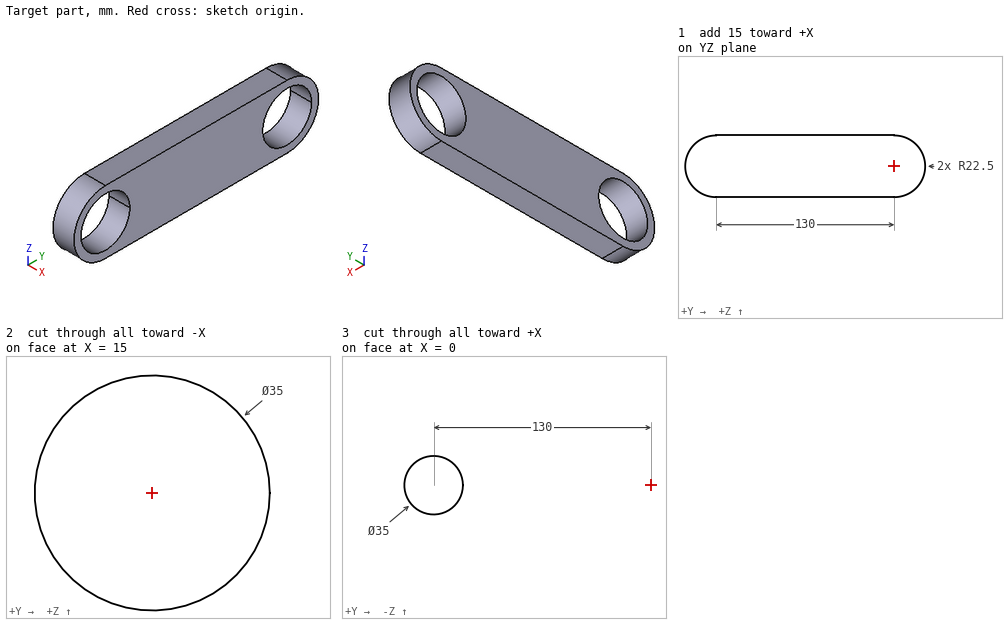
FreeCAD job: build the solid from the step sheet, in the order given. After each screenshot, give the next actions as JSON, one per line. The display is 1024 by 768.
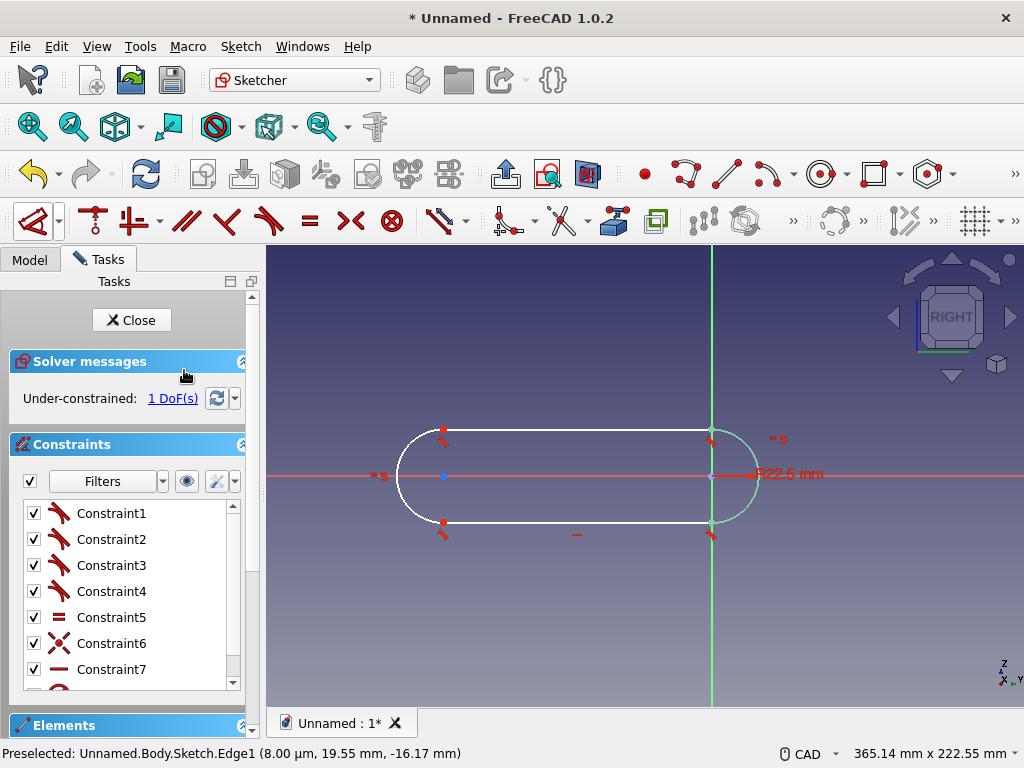
{"action": "left_click", "coordinate": [631, 523]}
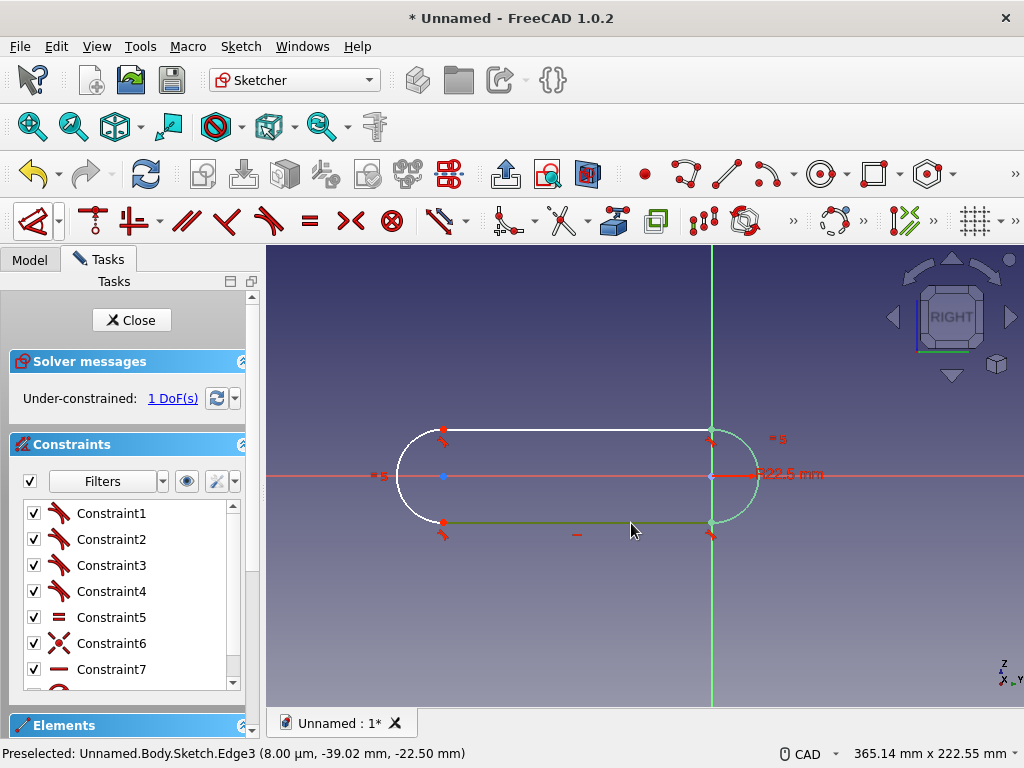
{"action": "left_click", "coordinate": [58, 222]}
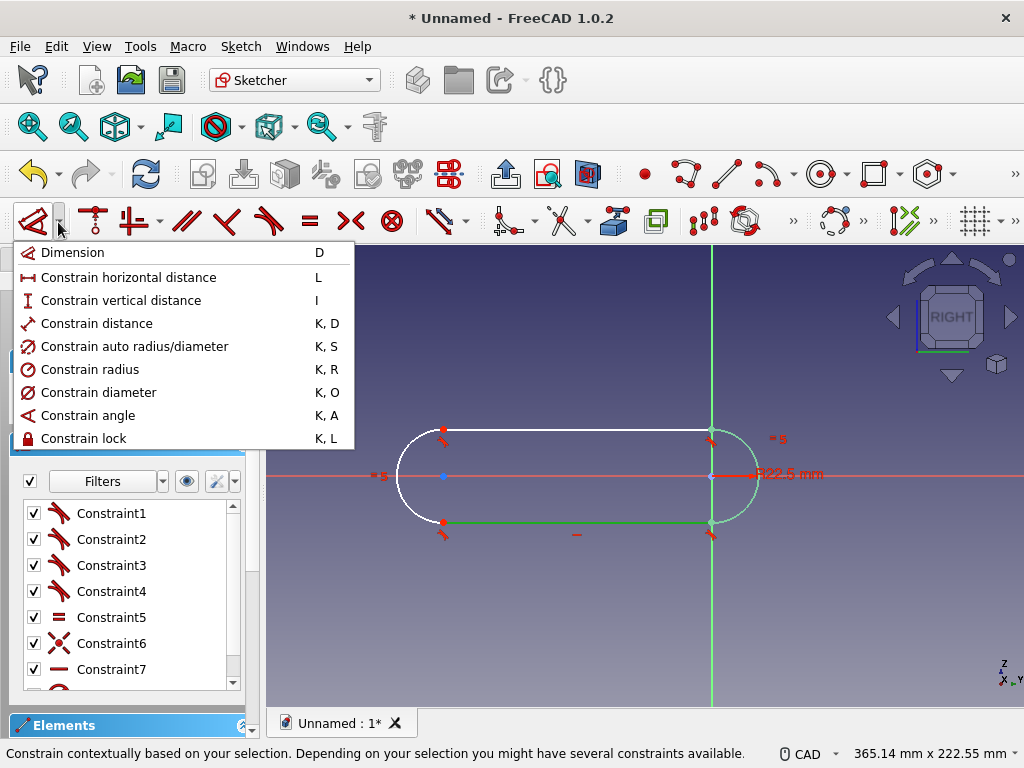
{"action": "left_click", "coordinate": [184, 278]}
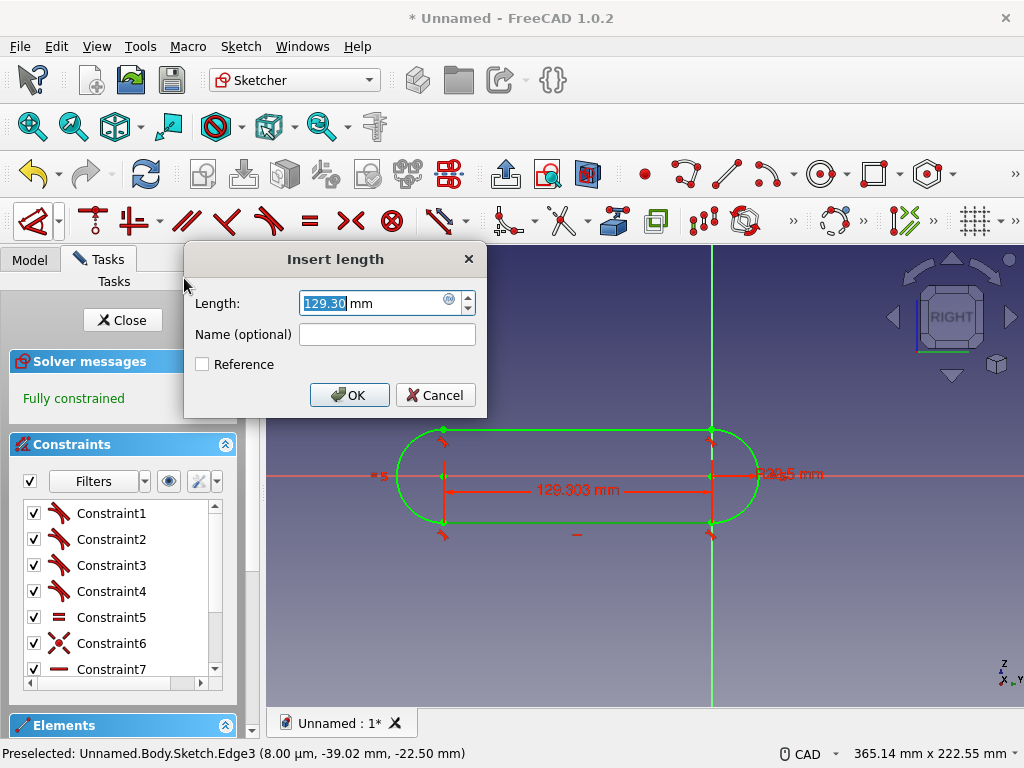
{"action": "type", "text": "130"}
{"action": "key", "text": "Return"}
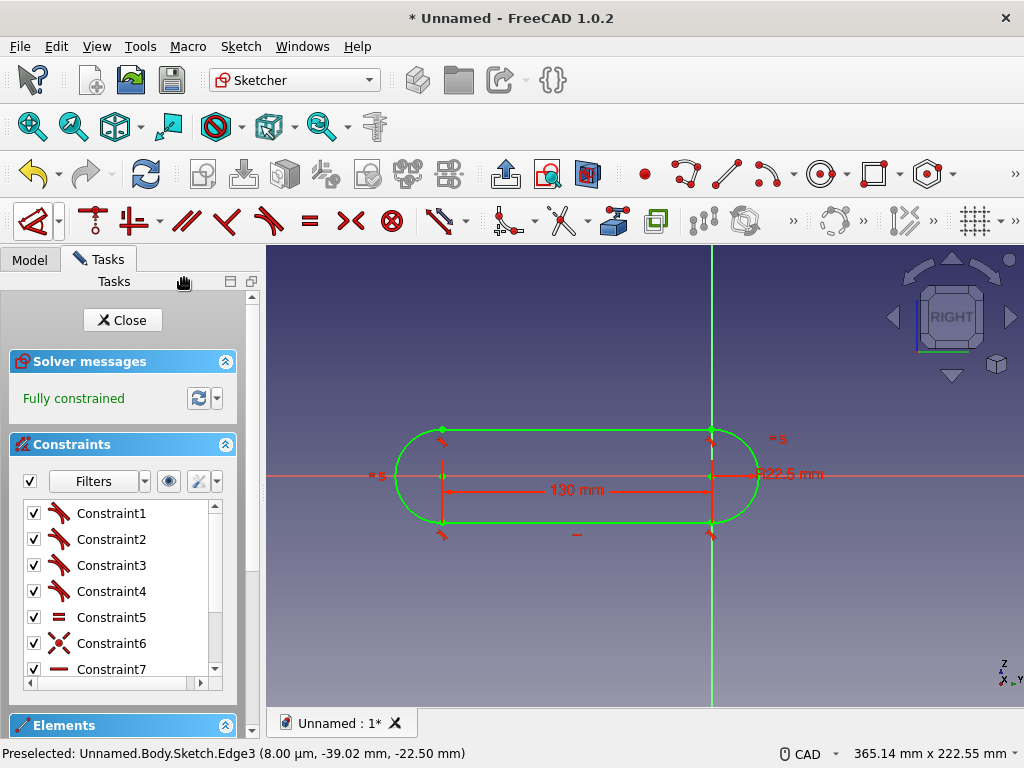
{"action": "left_click", "coordinate": [123, 320]}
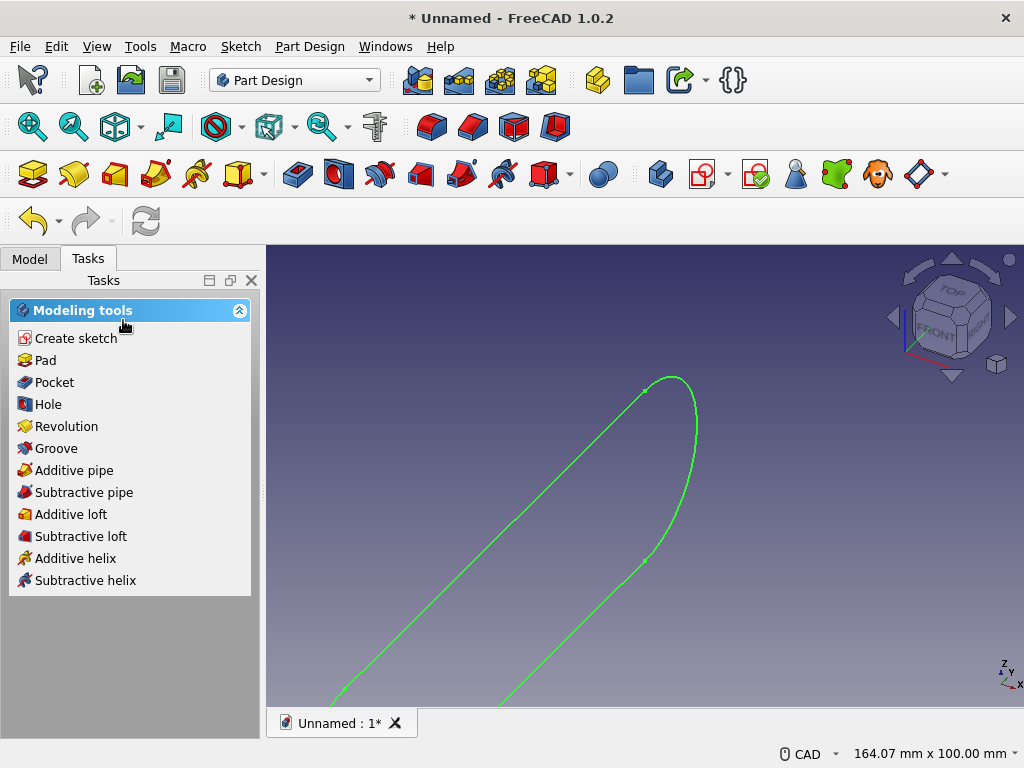
{"action": "left_click", "coordinate": [33, 174]}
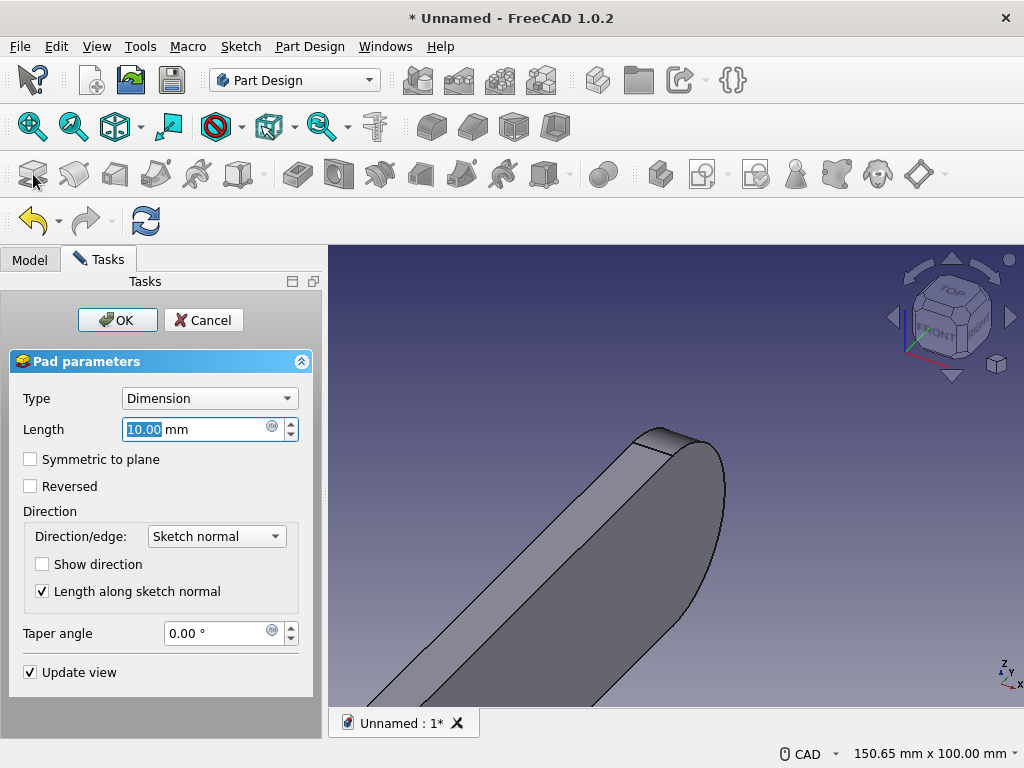
{"action": "type", "text": "15"}
{"action": "key", "text": "Tab"}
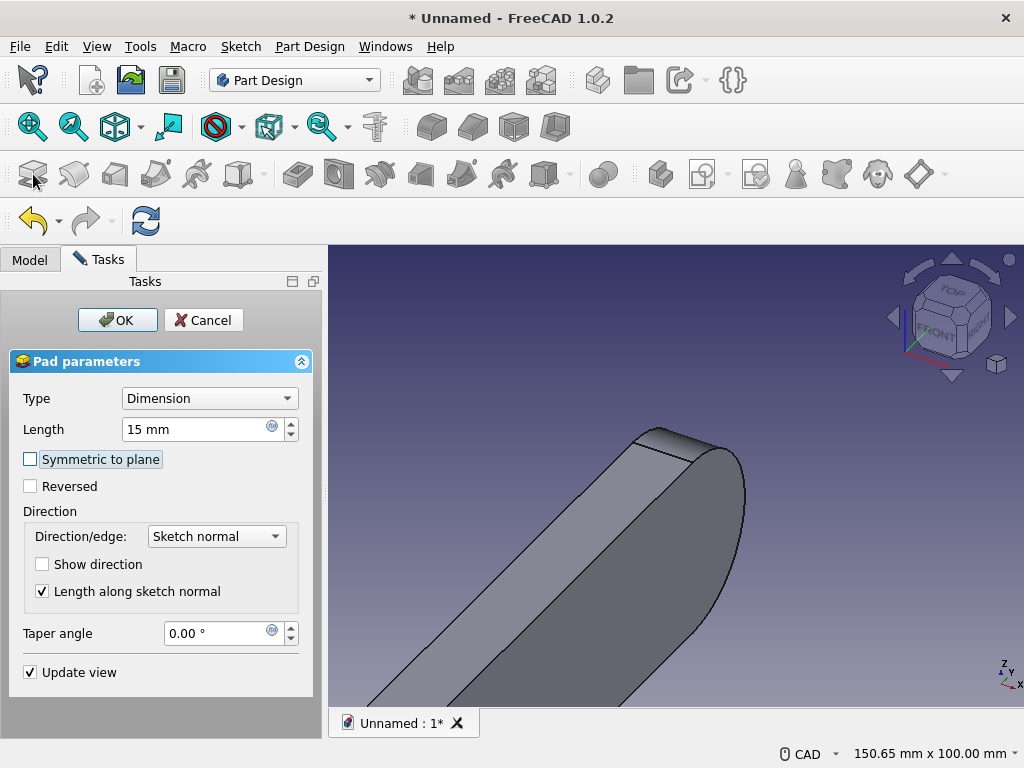
{"action": "left_click", "coordinate": [118, 320]}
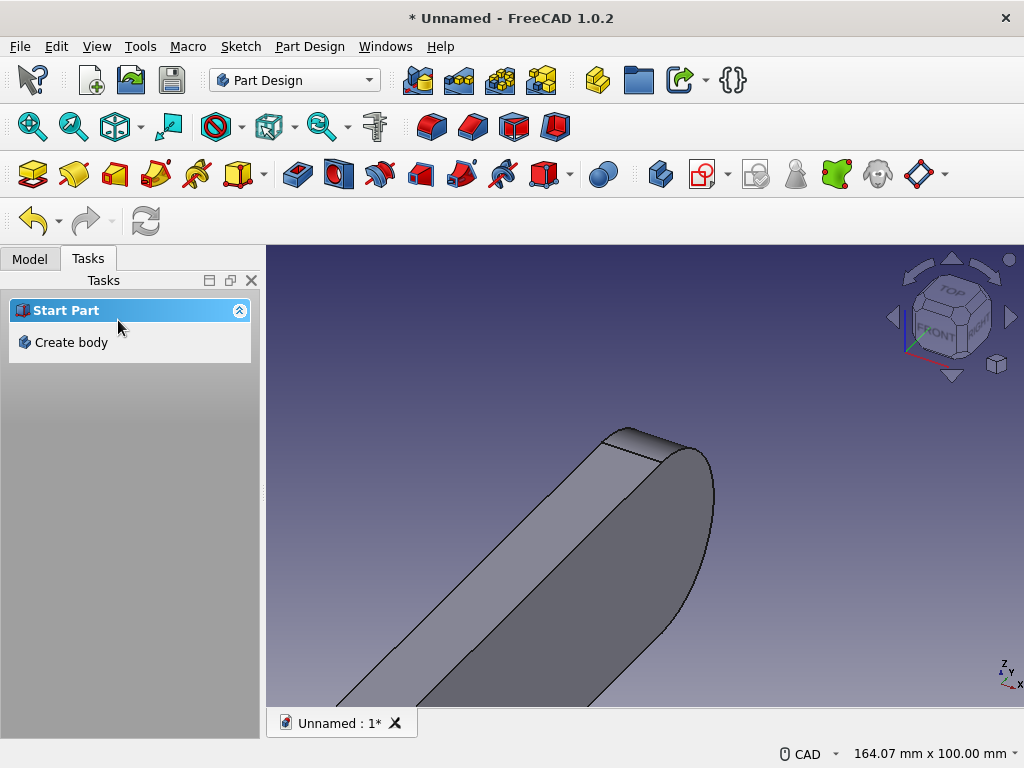
{"action": "key", "text": "v f"}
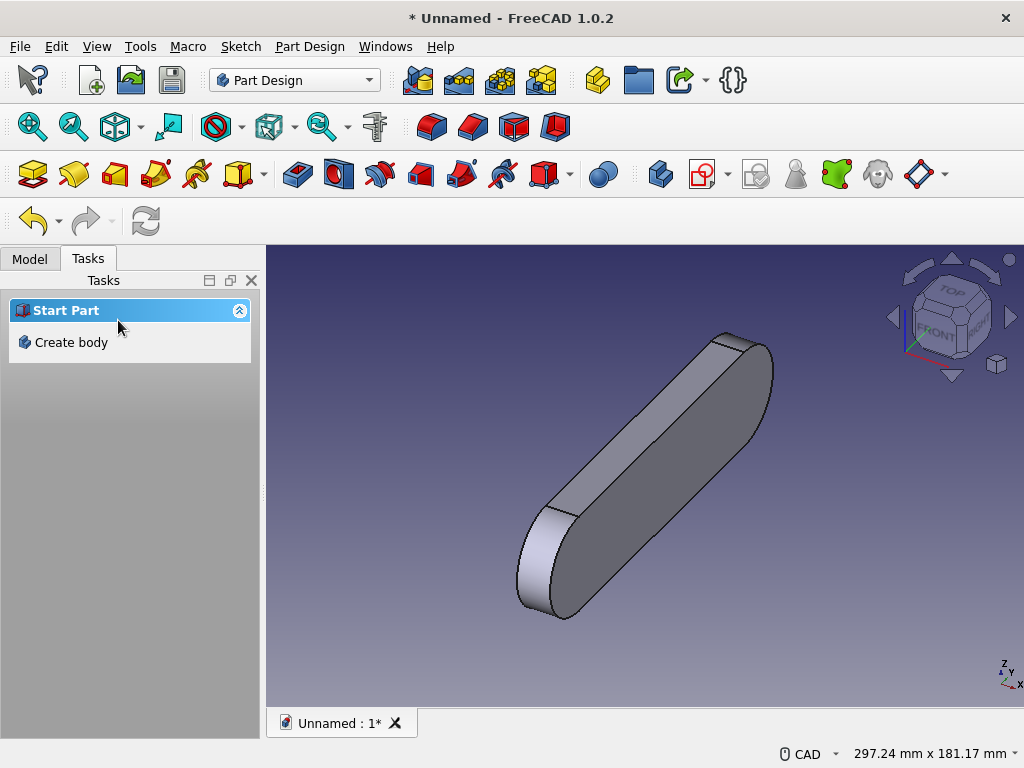
{"action": "left_click", "coordinate": [725, 417]}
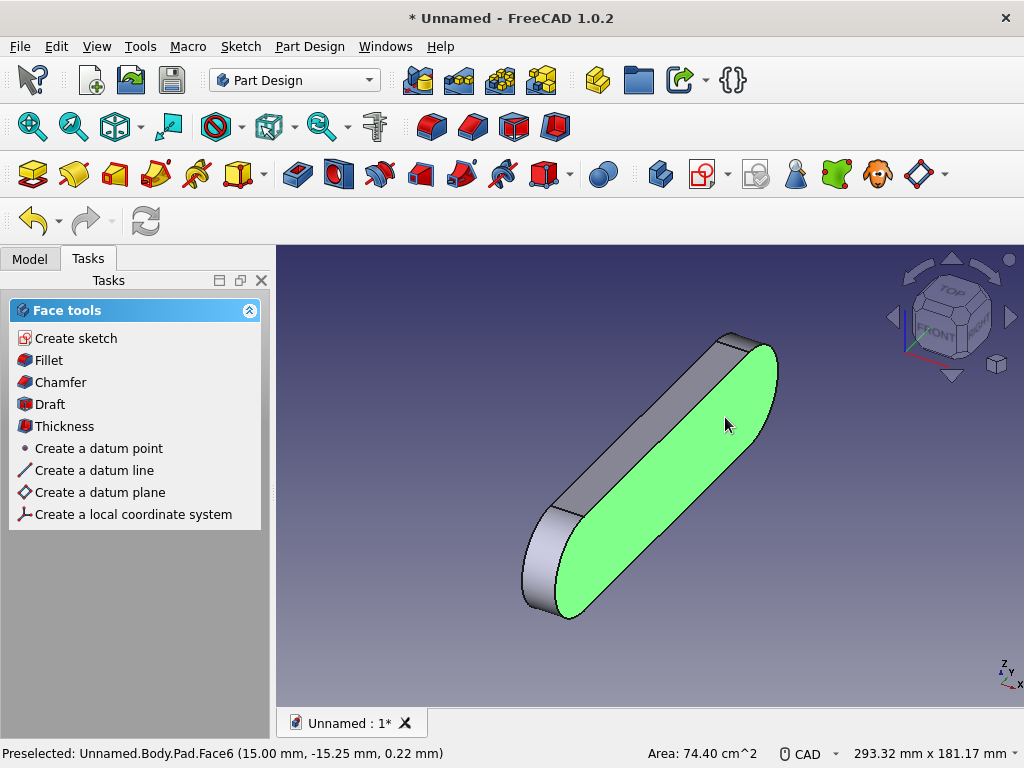
{"action": "left_click", "coordinate": [702, 174]}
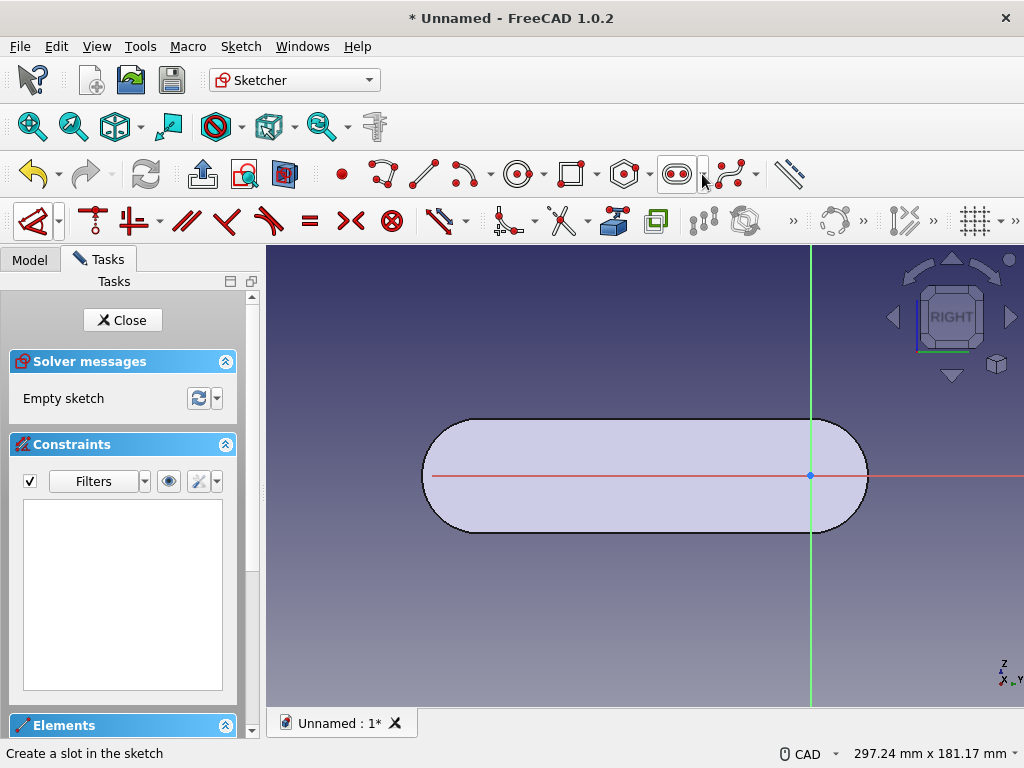
{"action": "scroll", "coordinate": [576, 476], "scroll_direction": "down", "scroll_amount": 5}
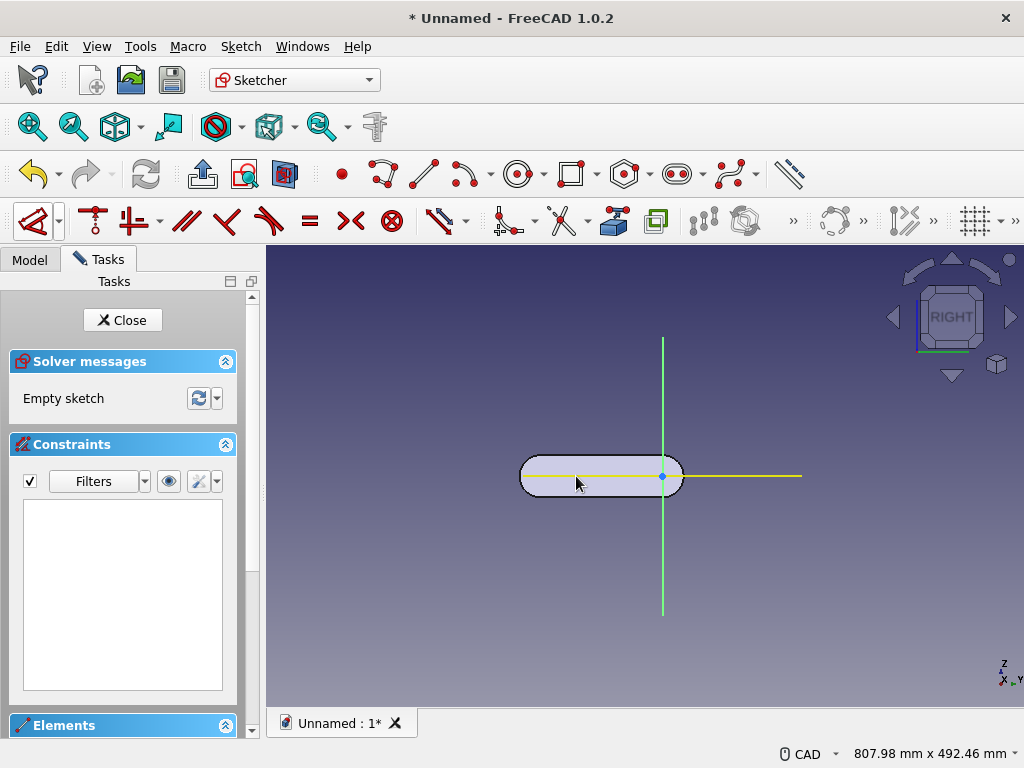
{"action": "scroll", "coordinate": [673, 476], "scroll_direction": "up", "scroll_amount": 11}